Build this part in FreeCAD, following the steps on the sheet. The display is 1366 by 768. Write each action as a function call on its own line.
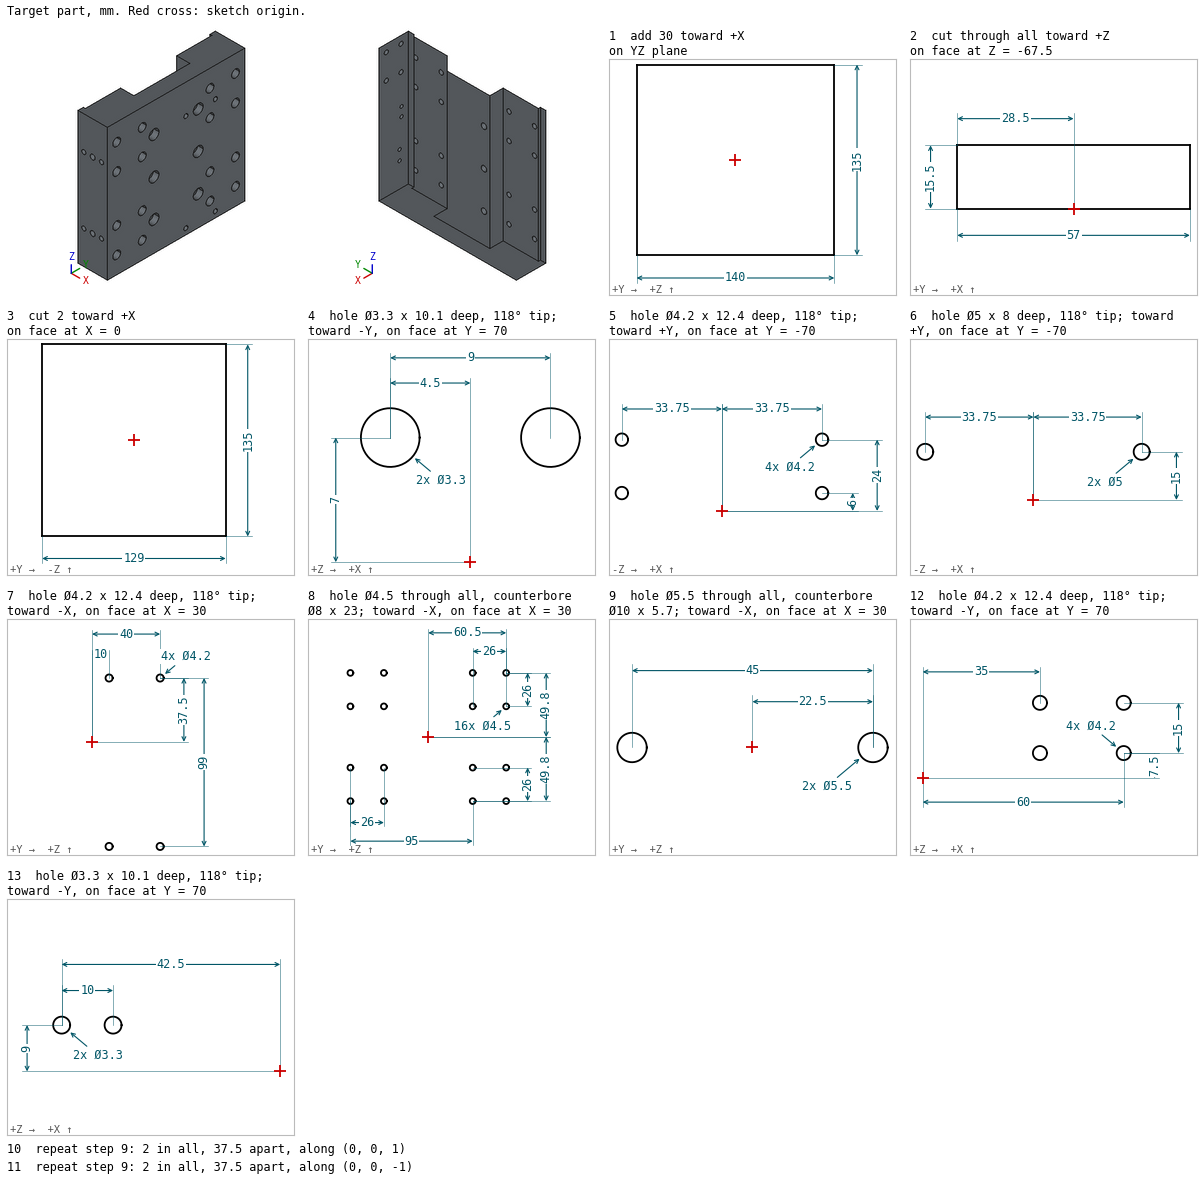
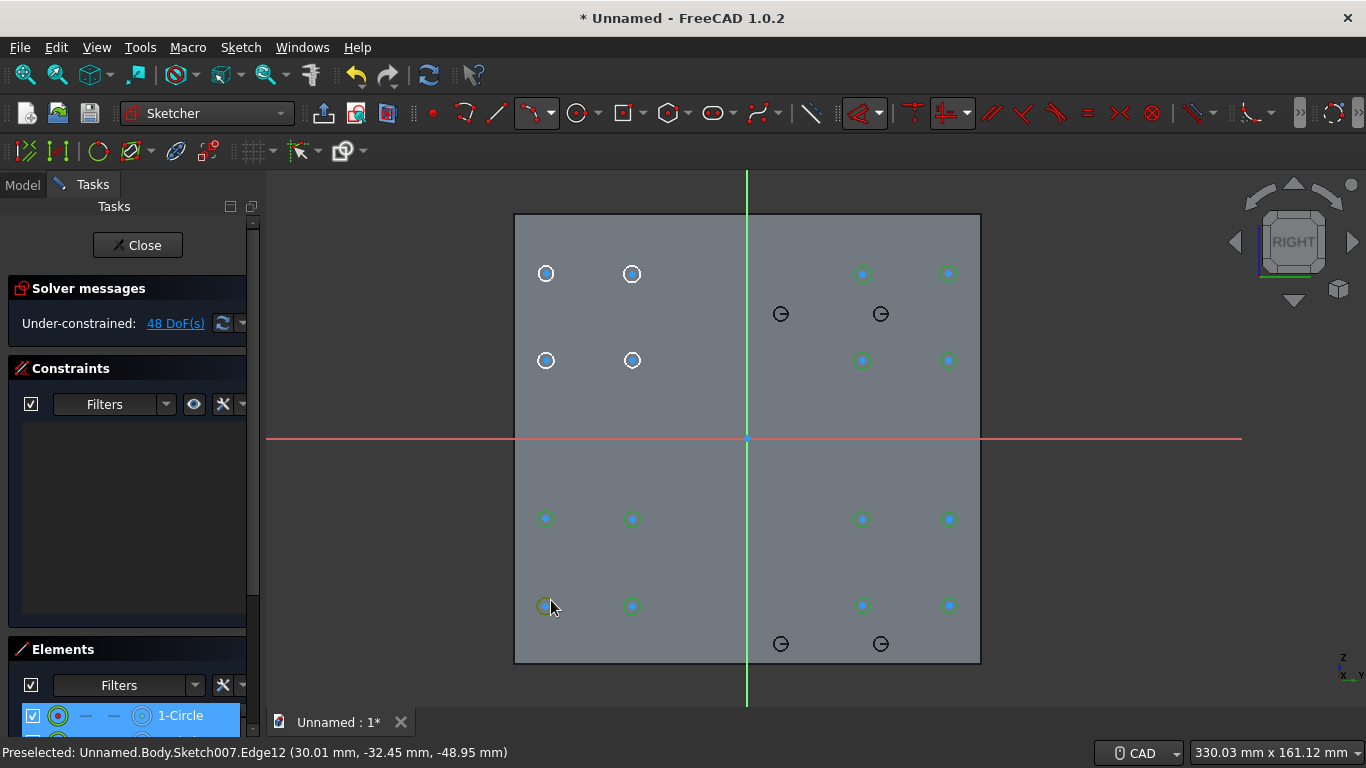
scroll(638, 268, up, 3)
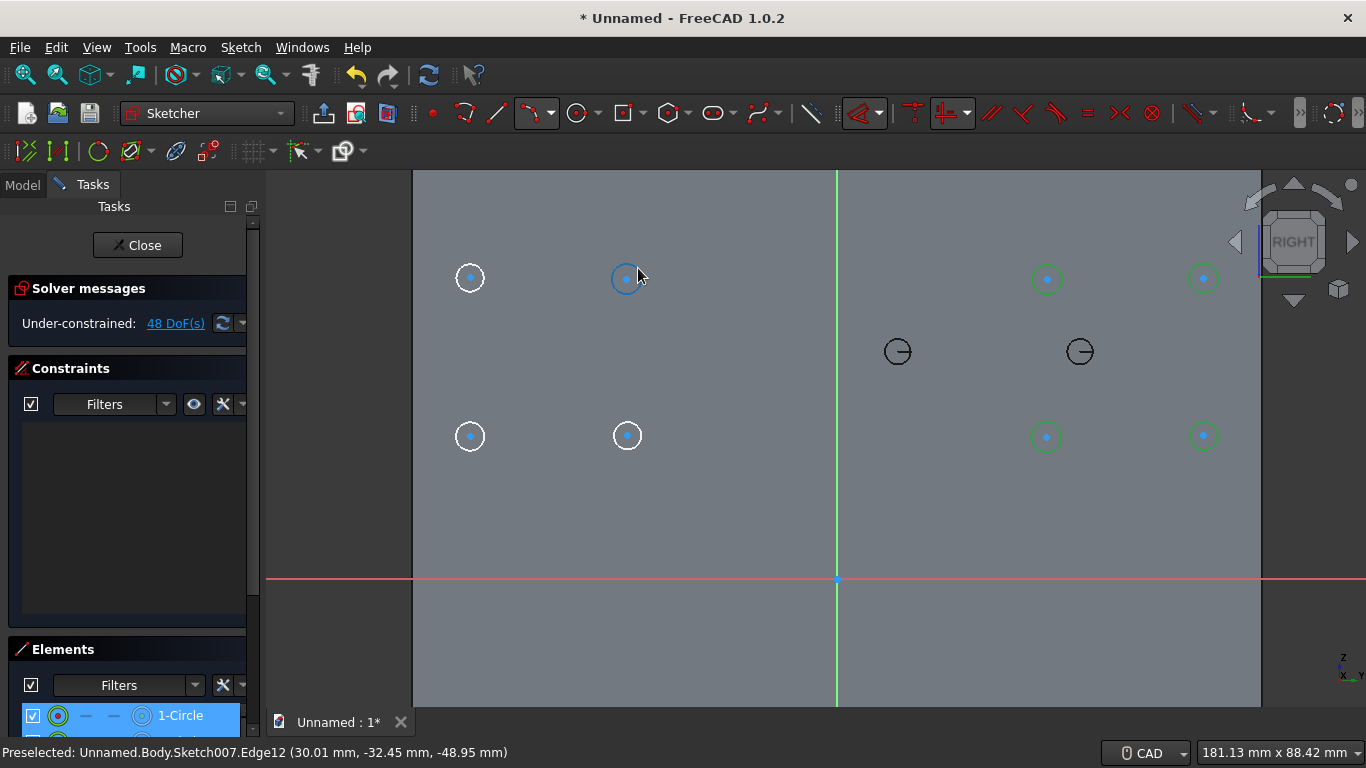
click(637, 268)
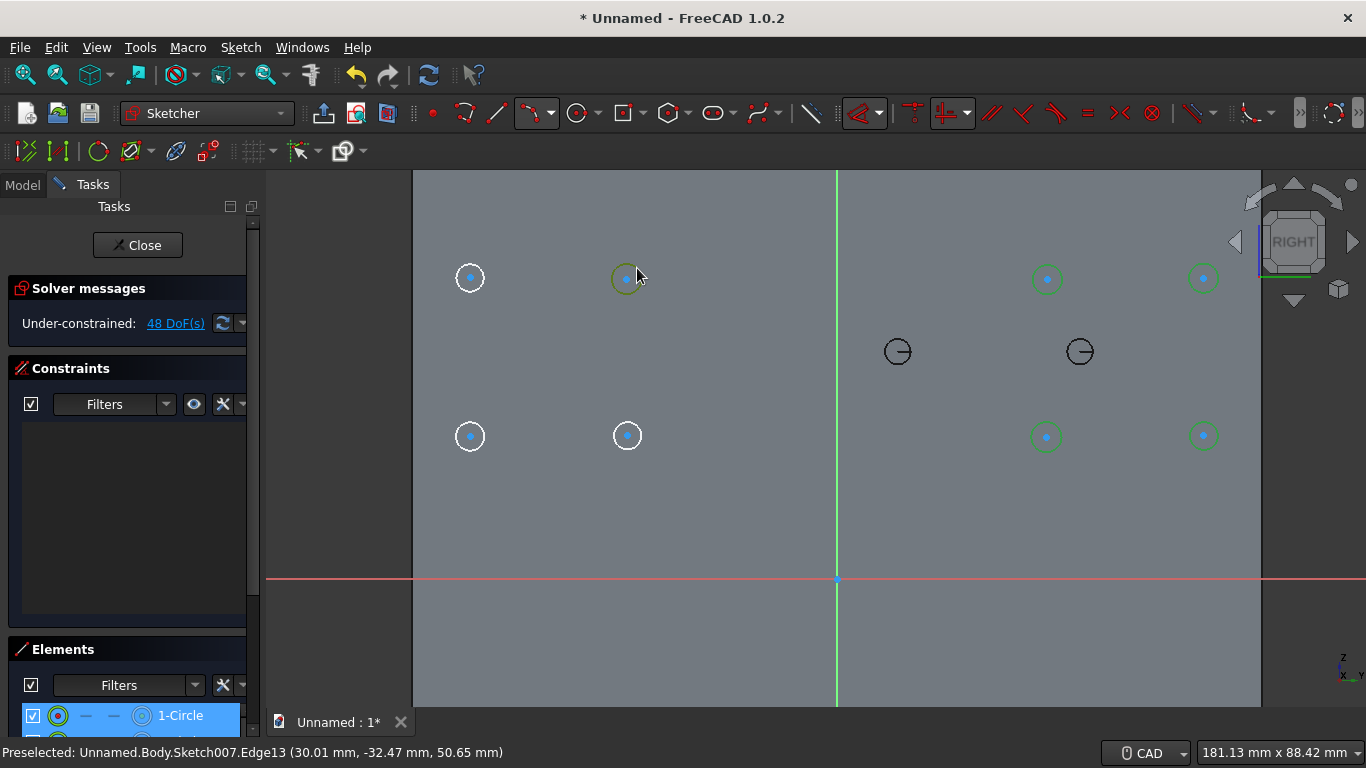
click(637, 426)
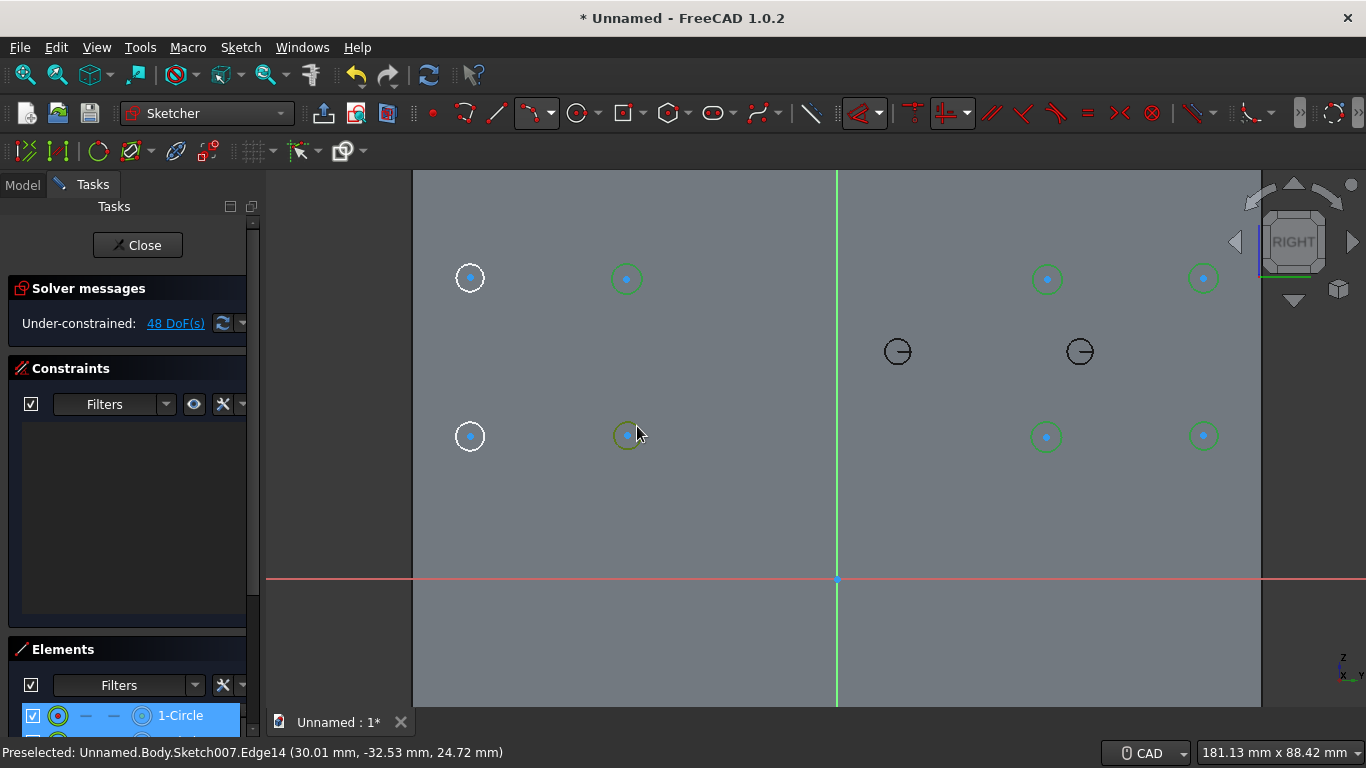
click(480, 426)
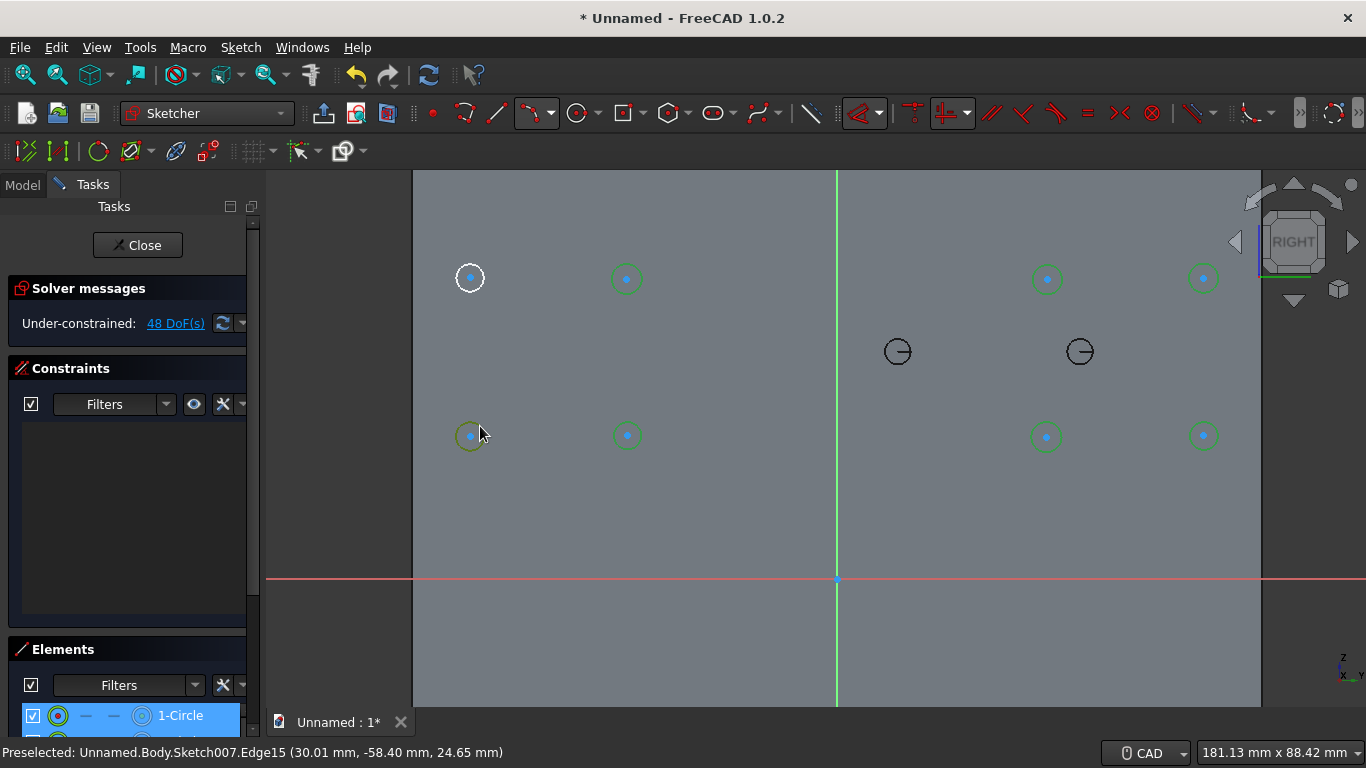
click(480, 268)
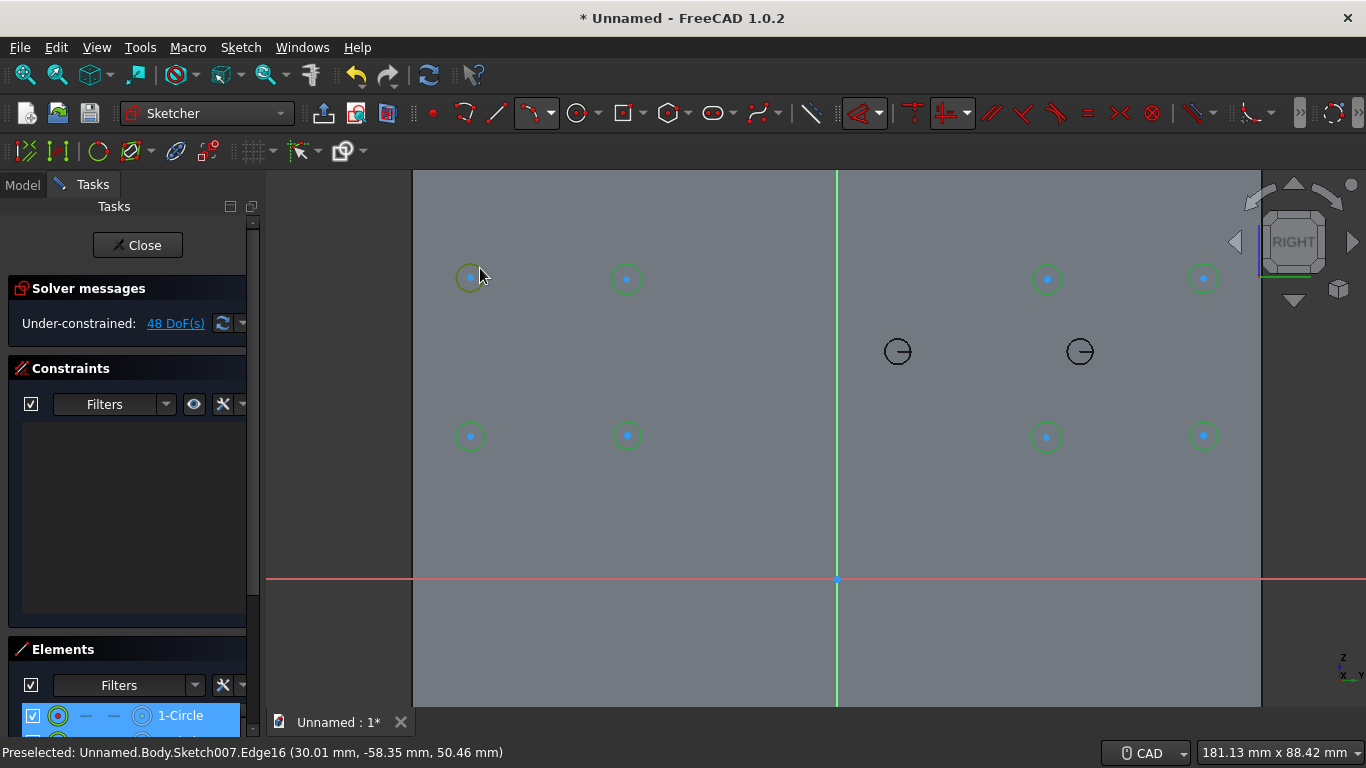
click(1088, 114)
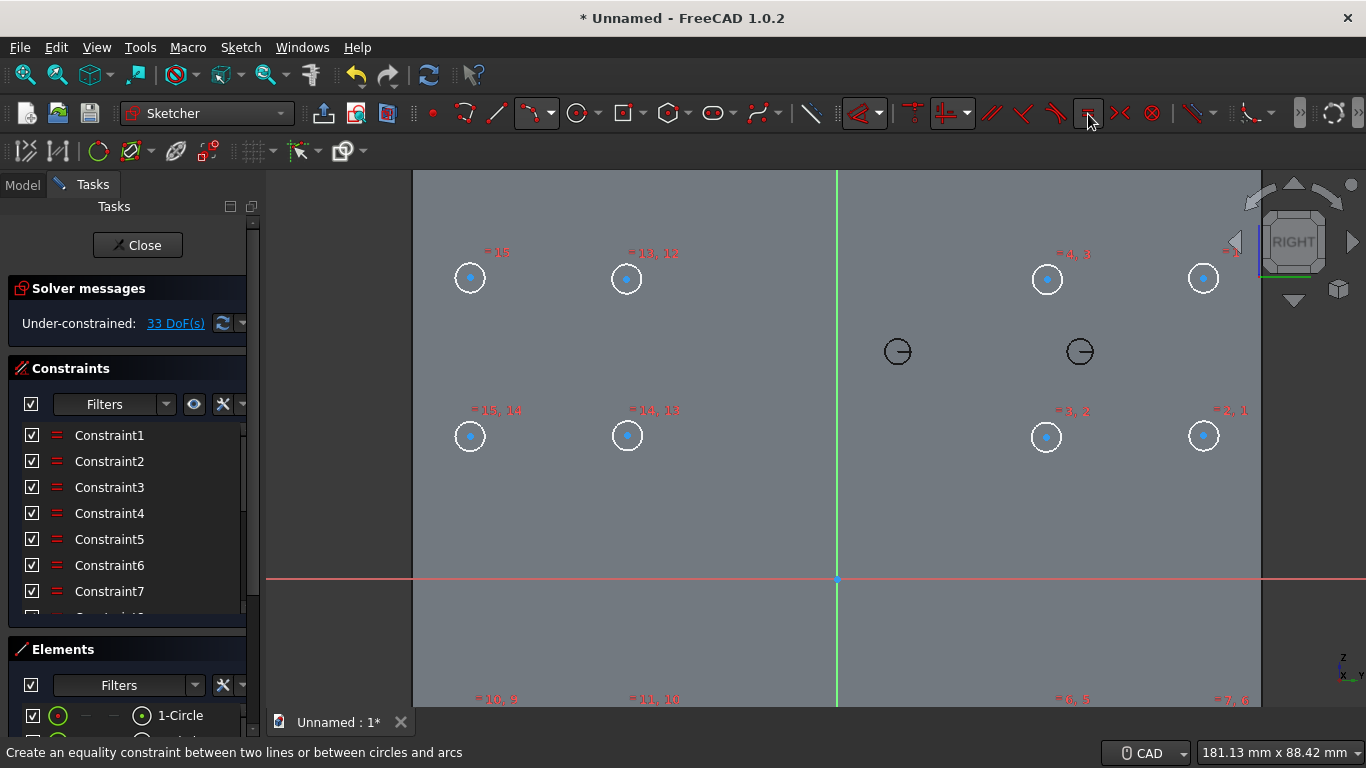
scroll(638, 267, down, 3)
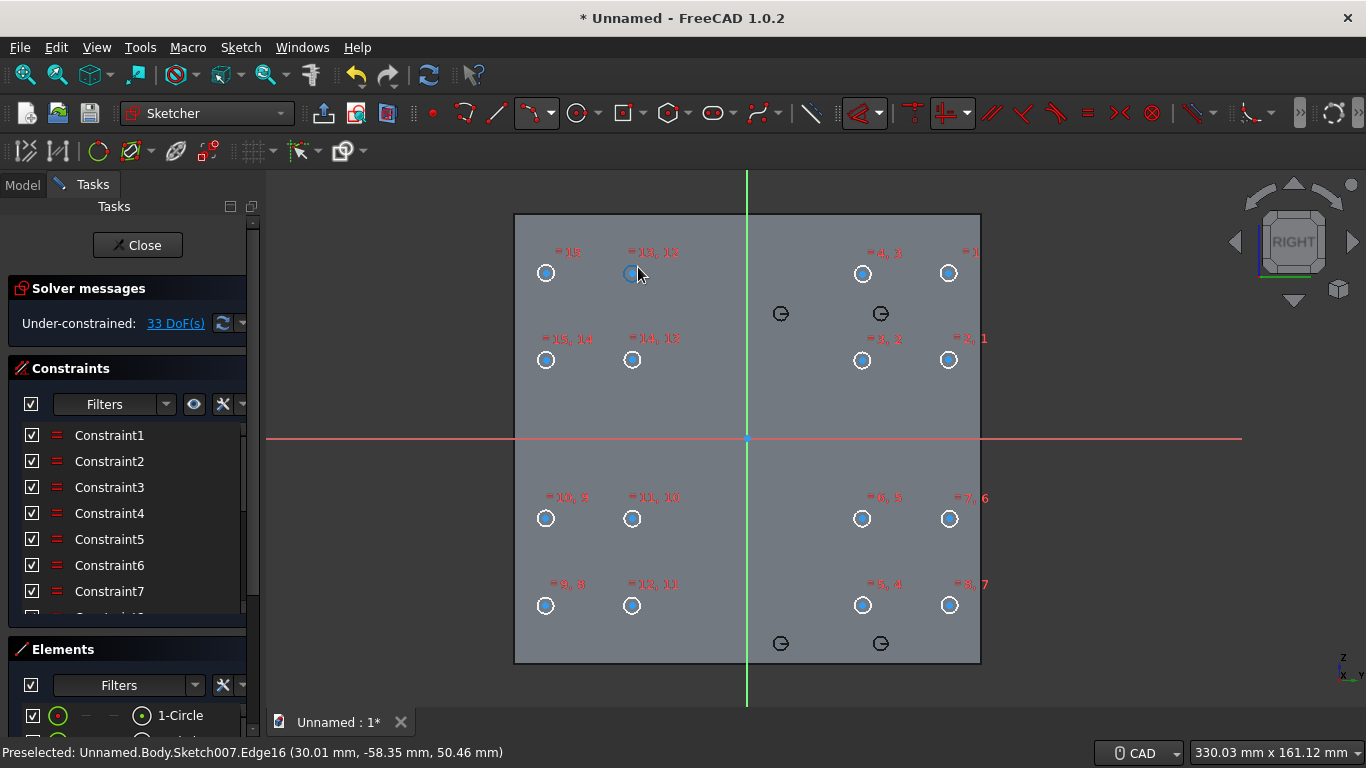
click(949, 273)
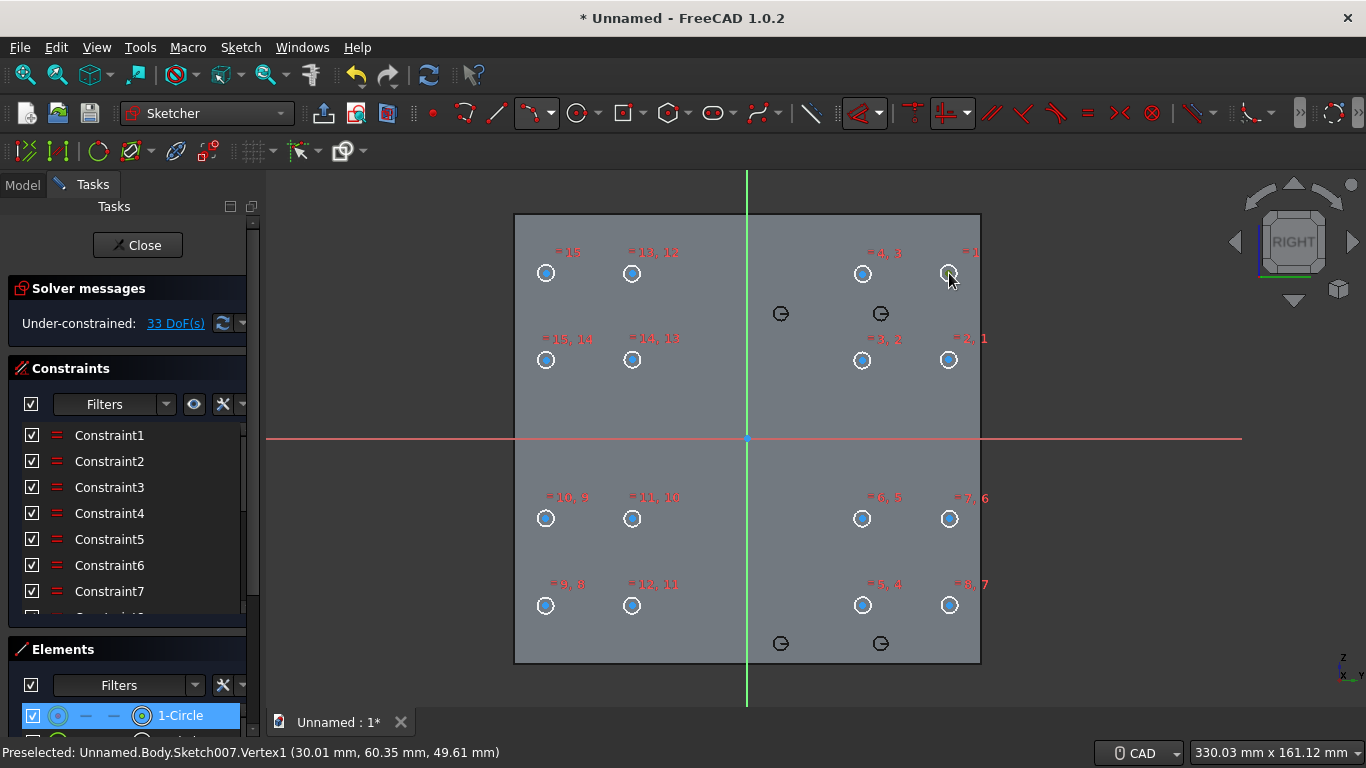
click(949, 360)